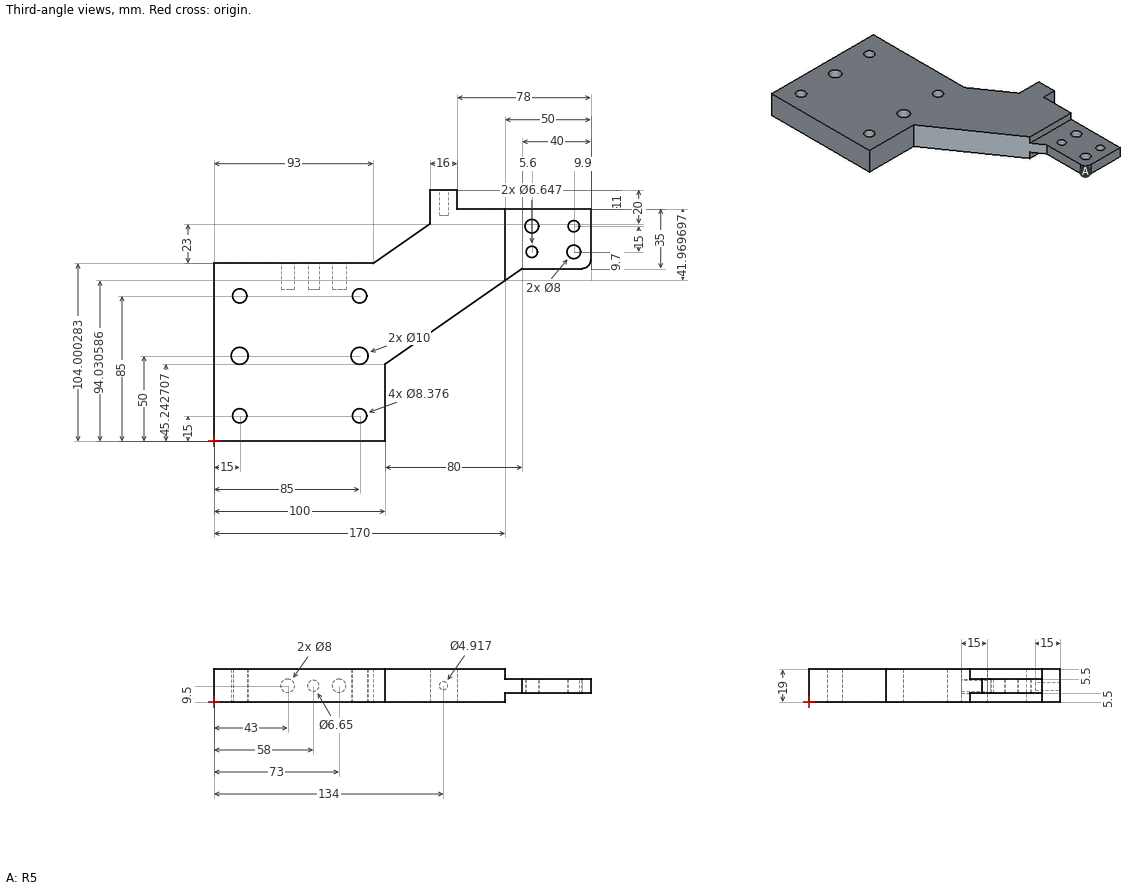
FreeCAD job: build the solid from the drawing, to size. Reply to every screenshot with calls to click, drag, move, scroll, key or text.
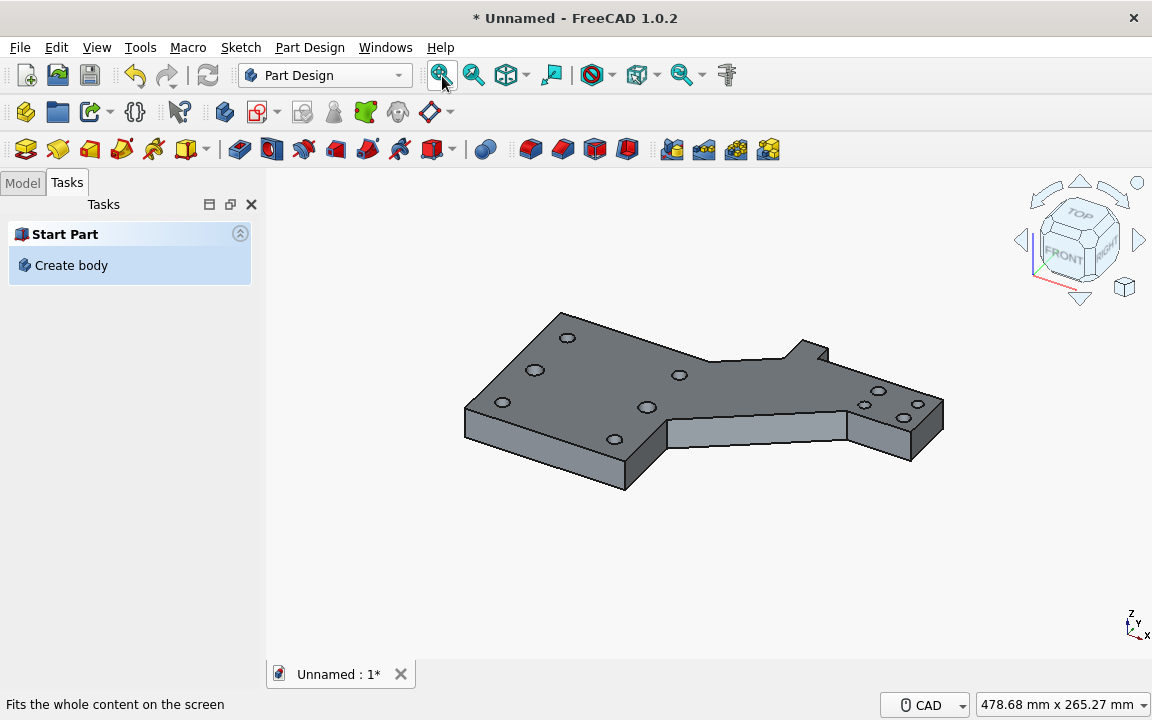
key(4)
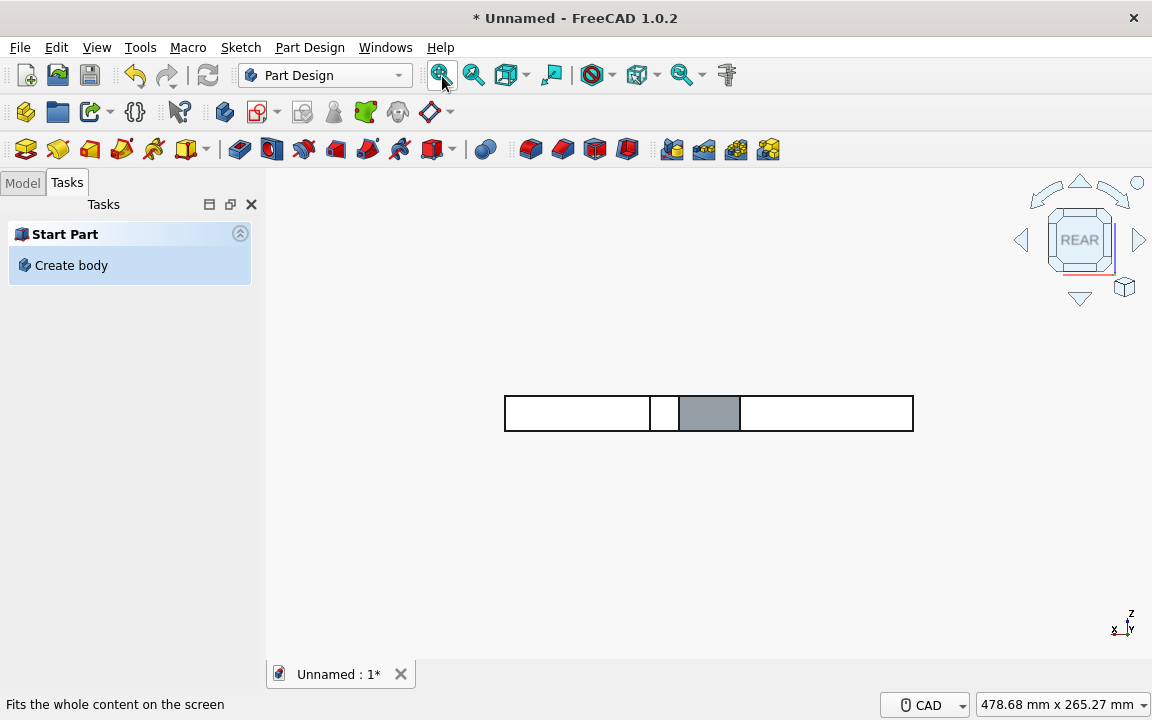
click(777, 413)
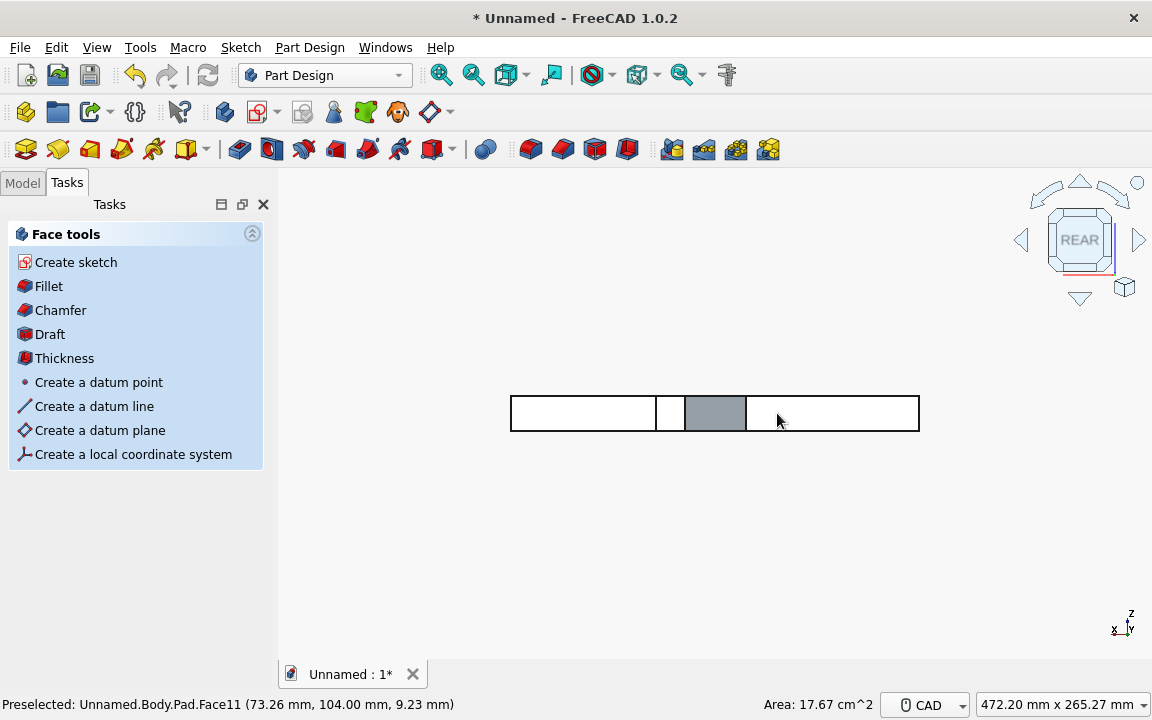
click(258, 112)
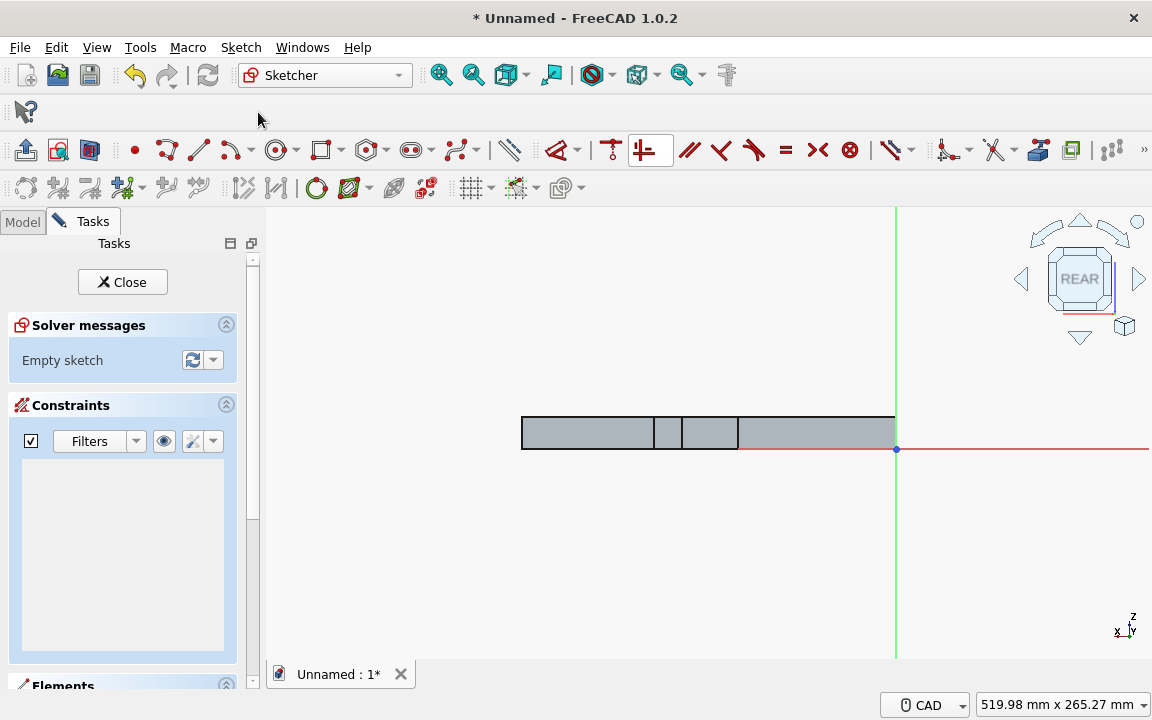
click(90, 150)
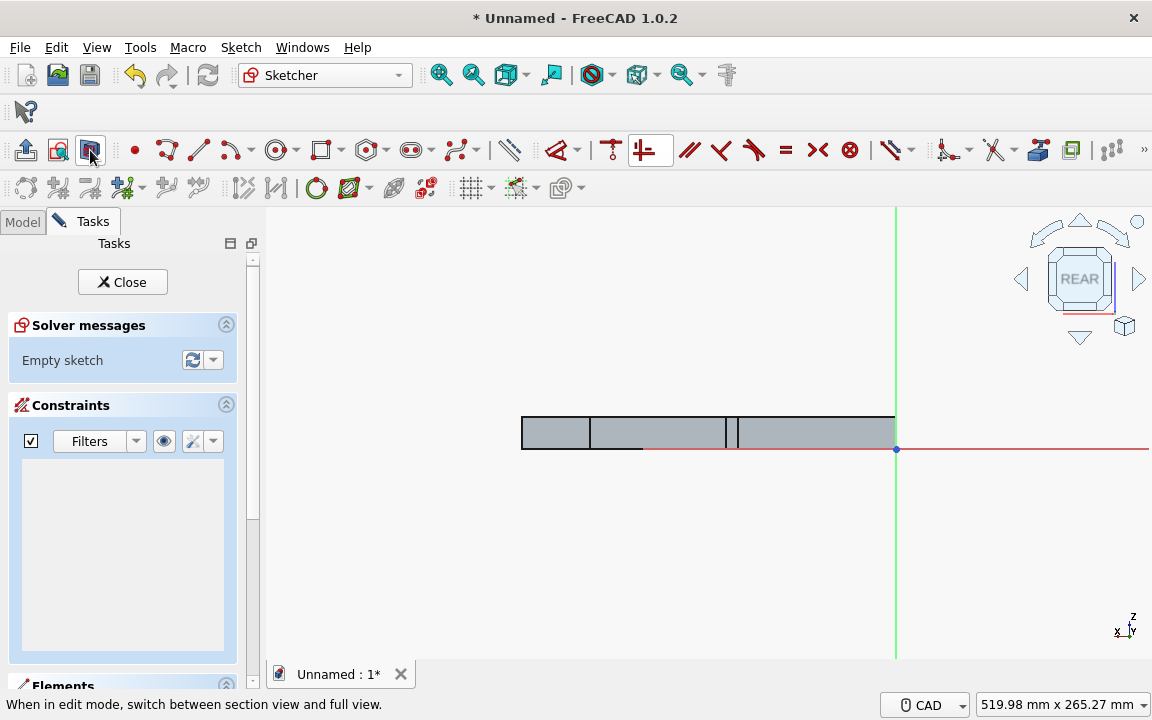
scroll(893, 439, up, 7)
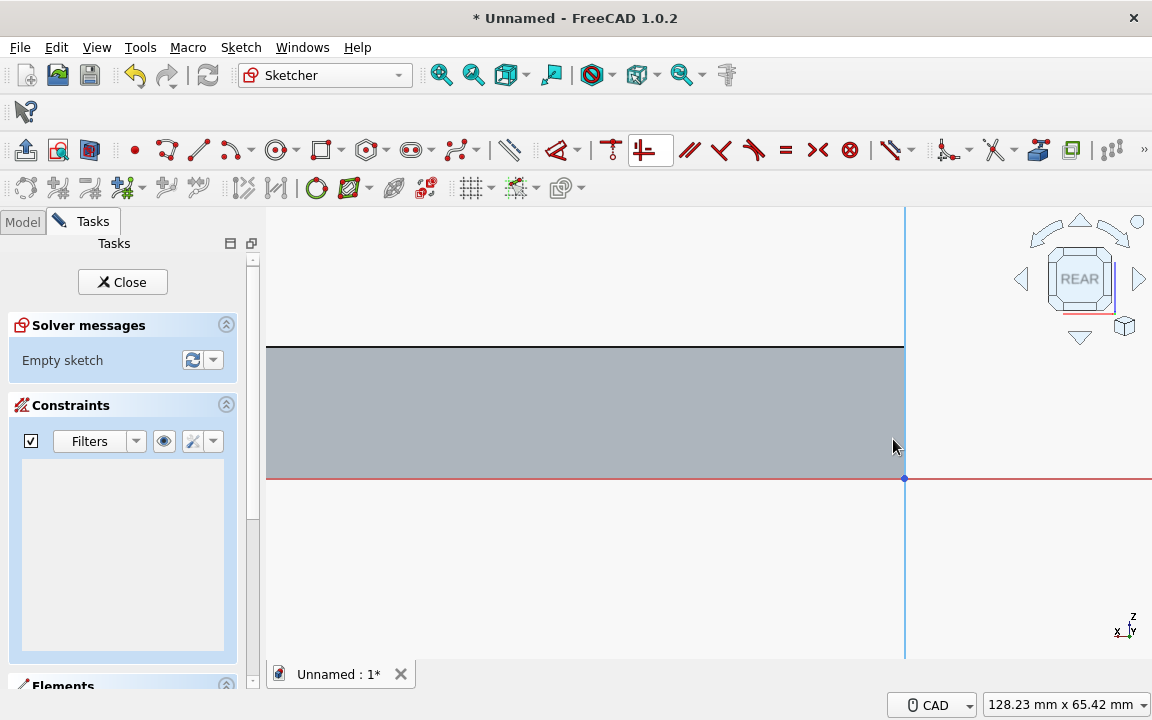
click(276, 150)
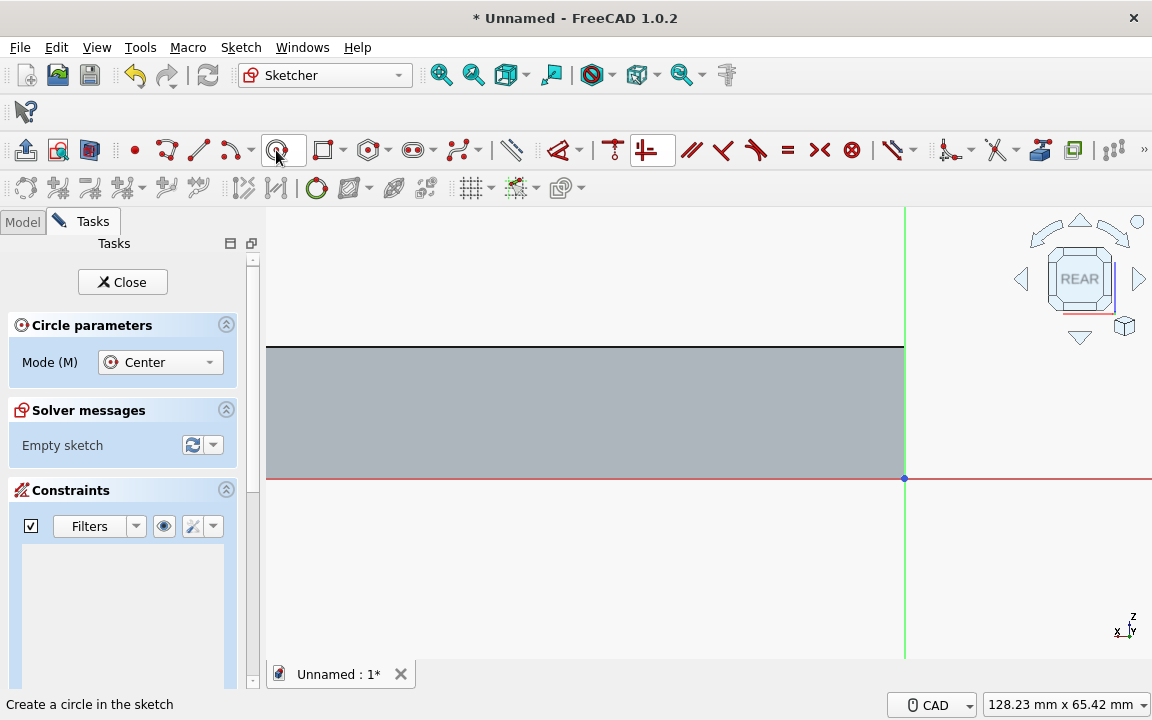
click(608, 413)
click(627, 394)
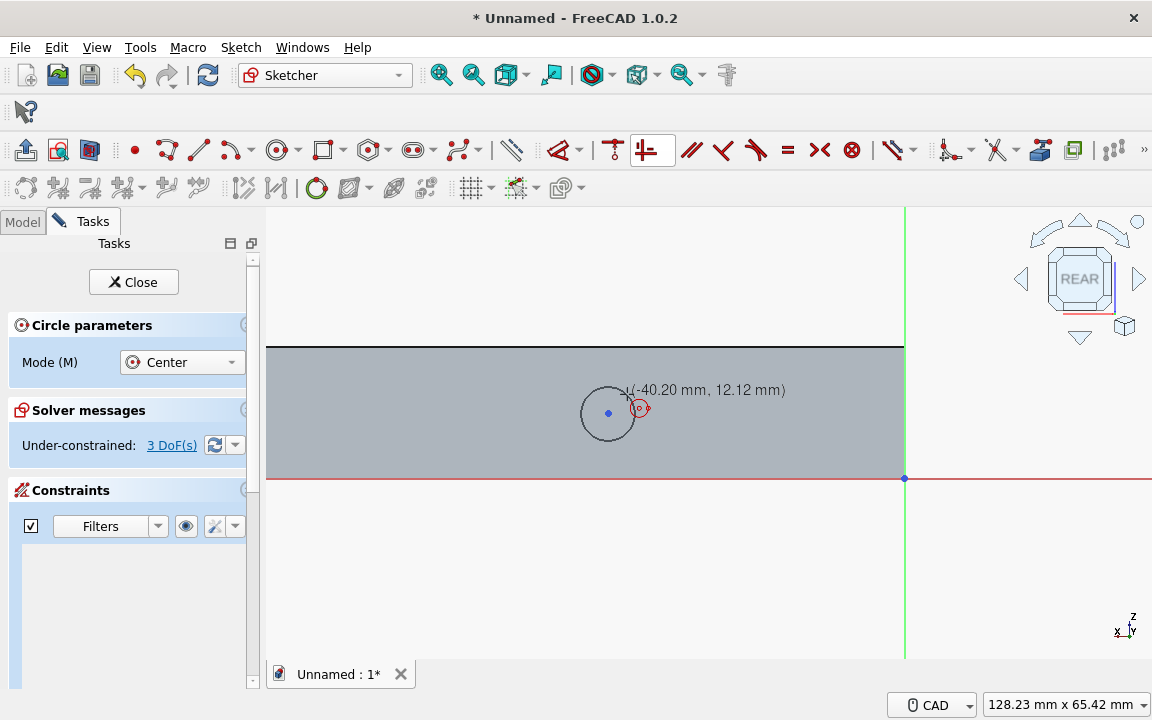
click(504, 413)
click(520, 397)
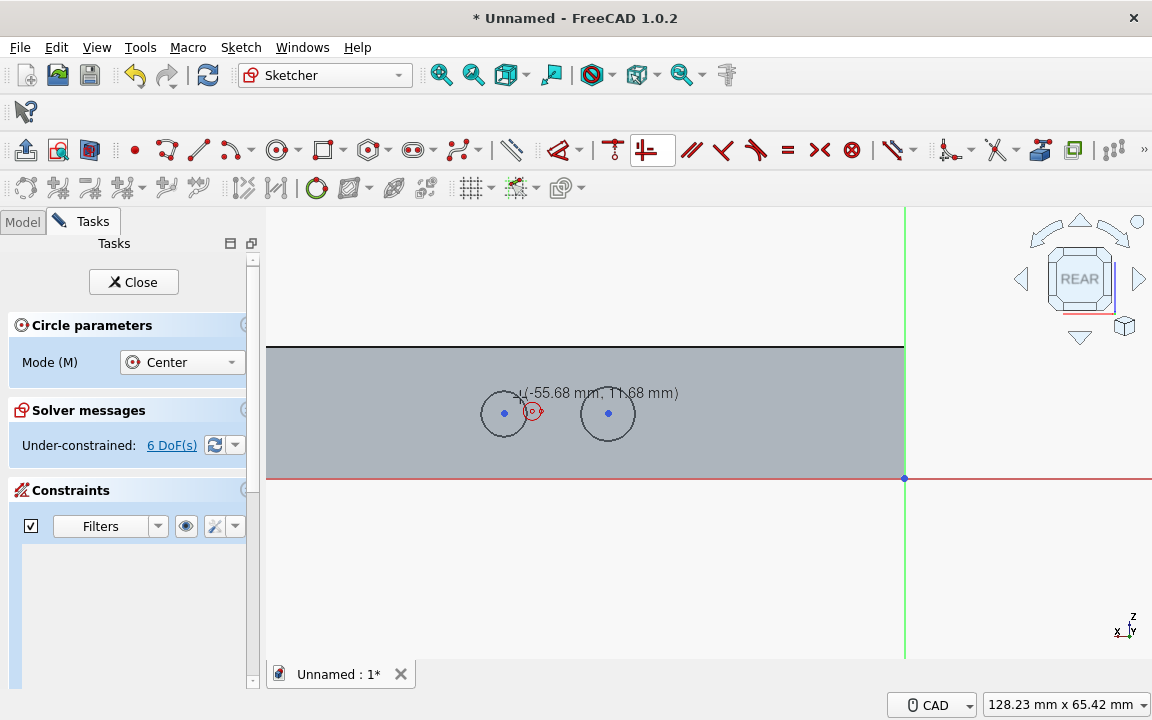
click(400, 413)
click(420, 394)
key(Escape)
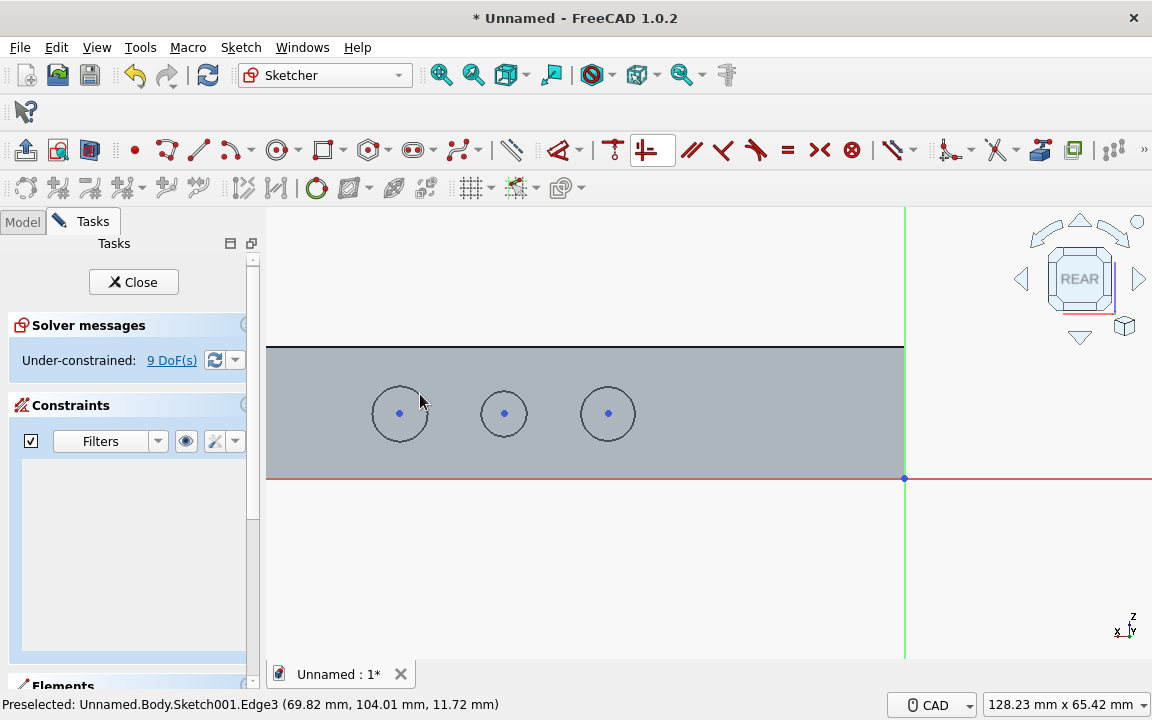
click(627, 395)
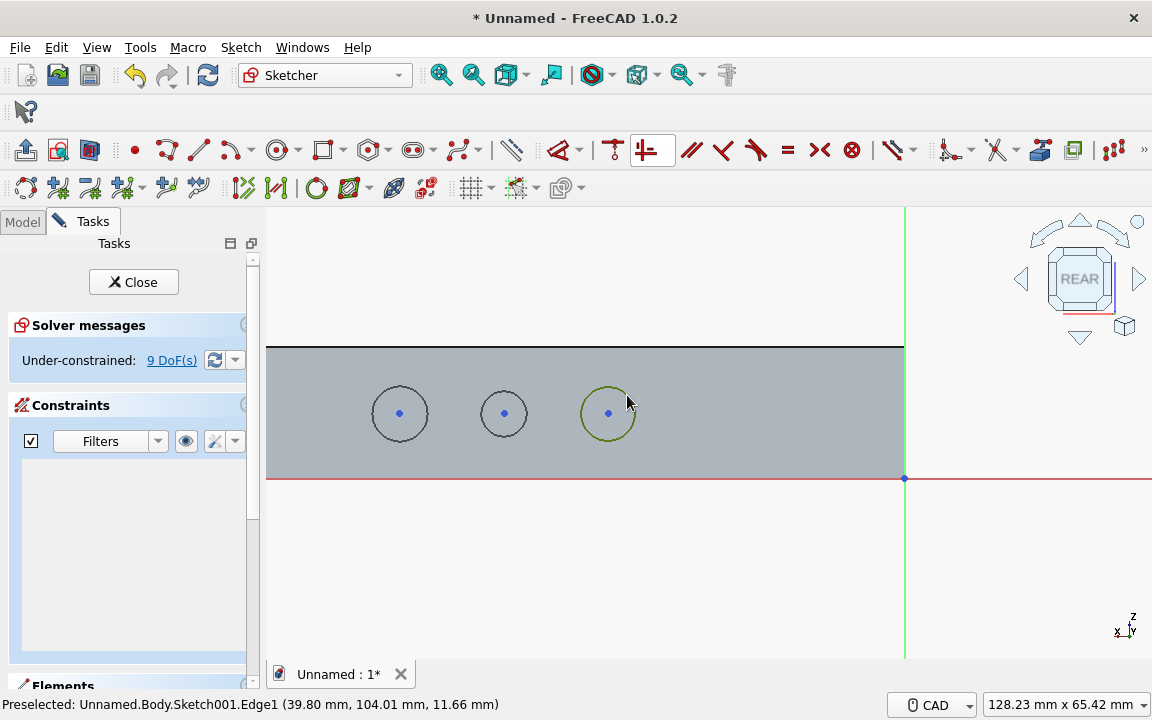
click(419, 394)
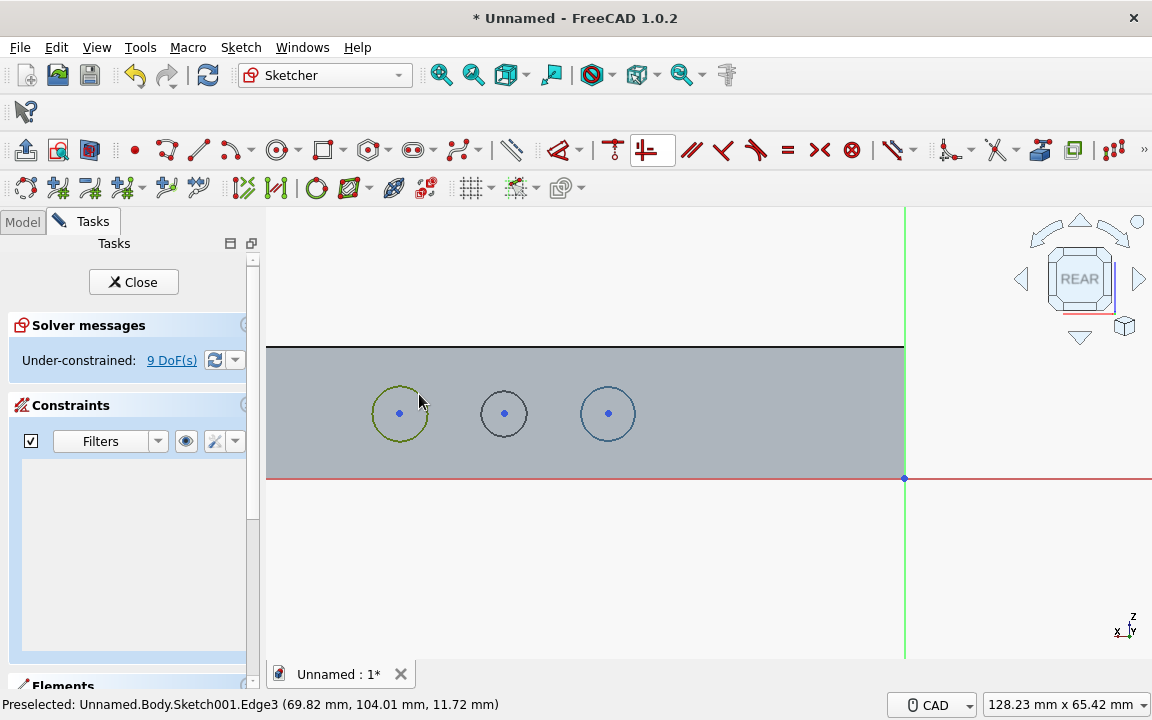
click(788, 150)